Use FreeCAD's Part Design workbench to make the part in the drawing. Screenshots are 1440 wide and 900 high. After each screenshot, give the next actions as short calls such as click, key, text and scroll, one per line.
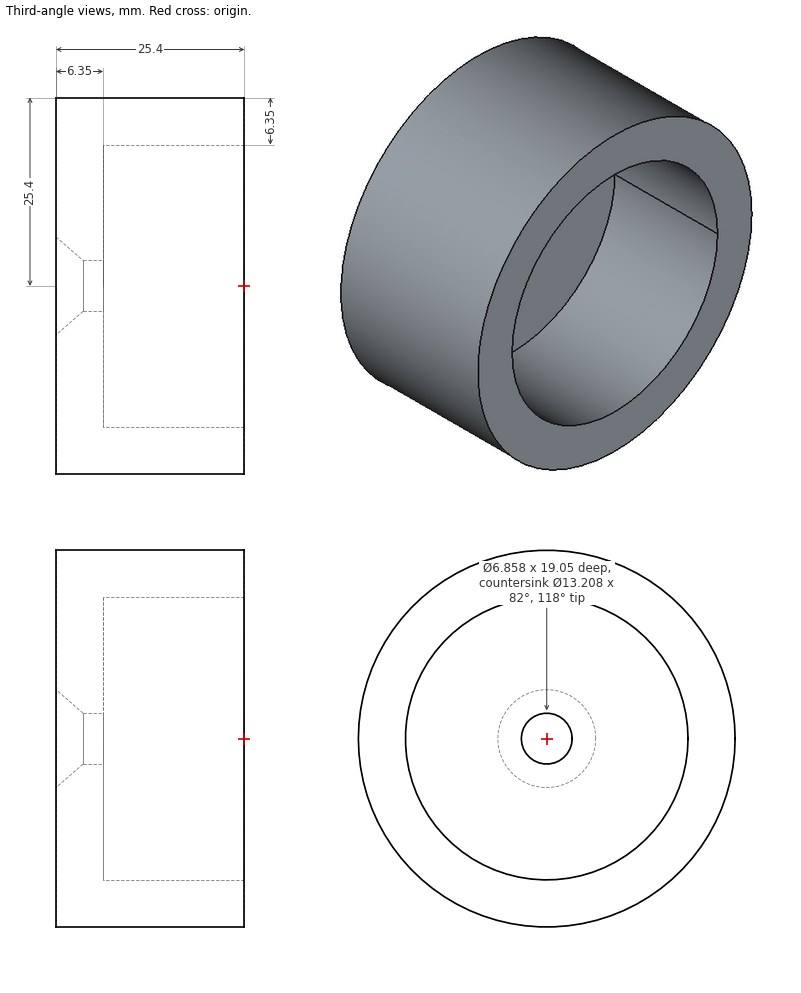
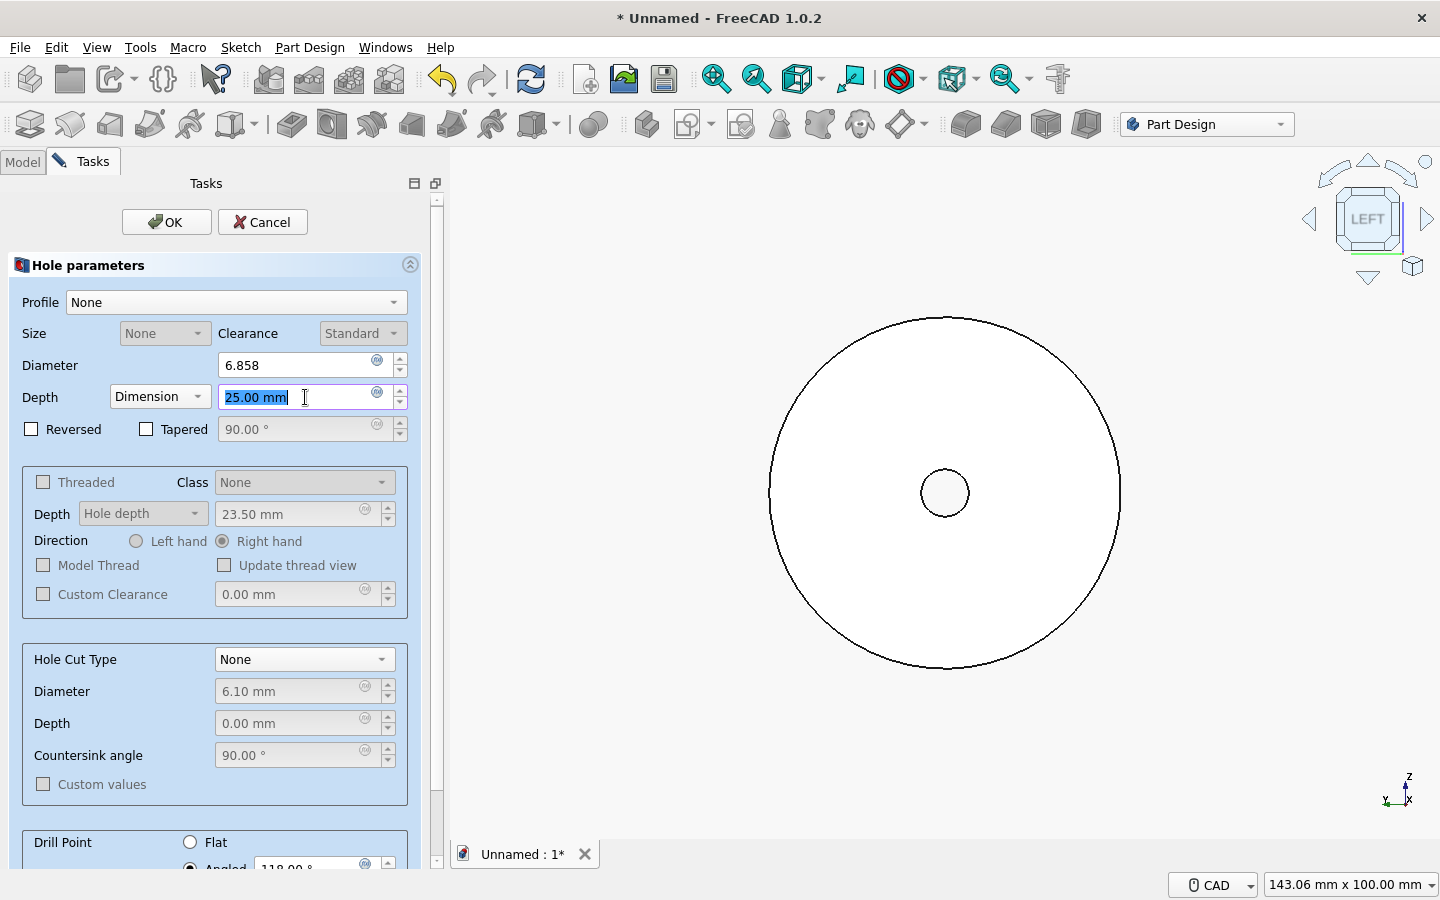
text(19.05)
key(Tab)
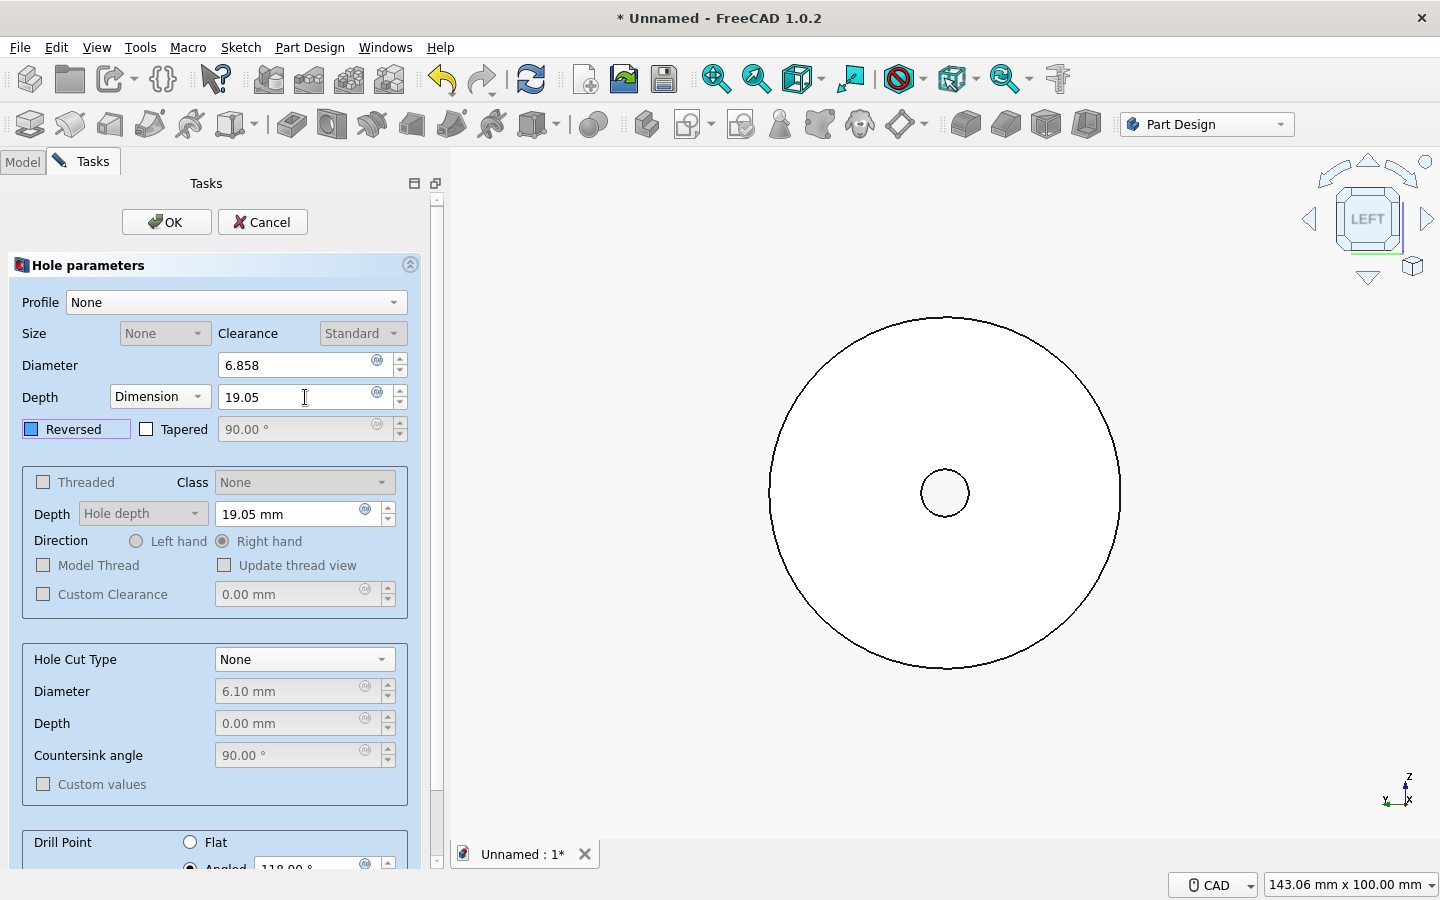
click(306, 660)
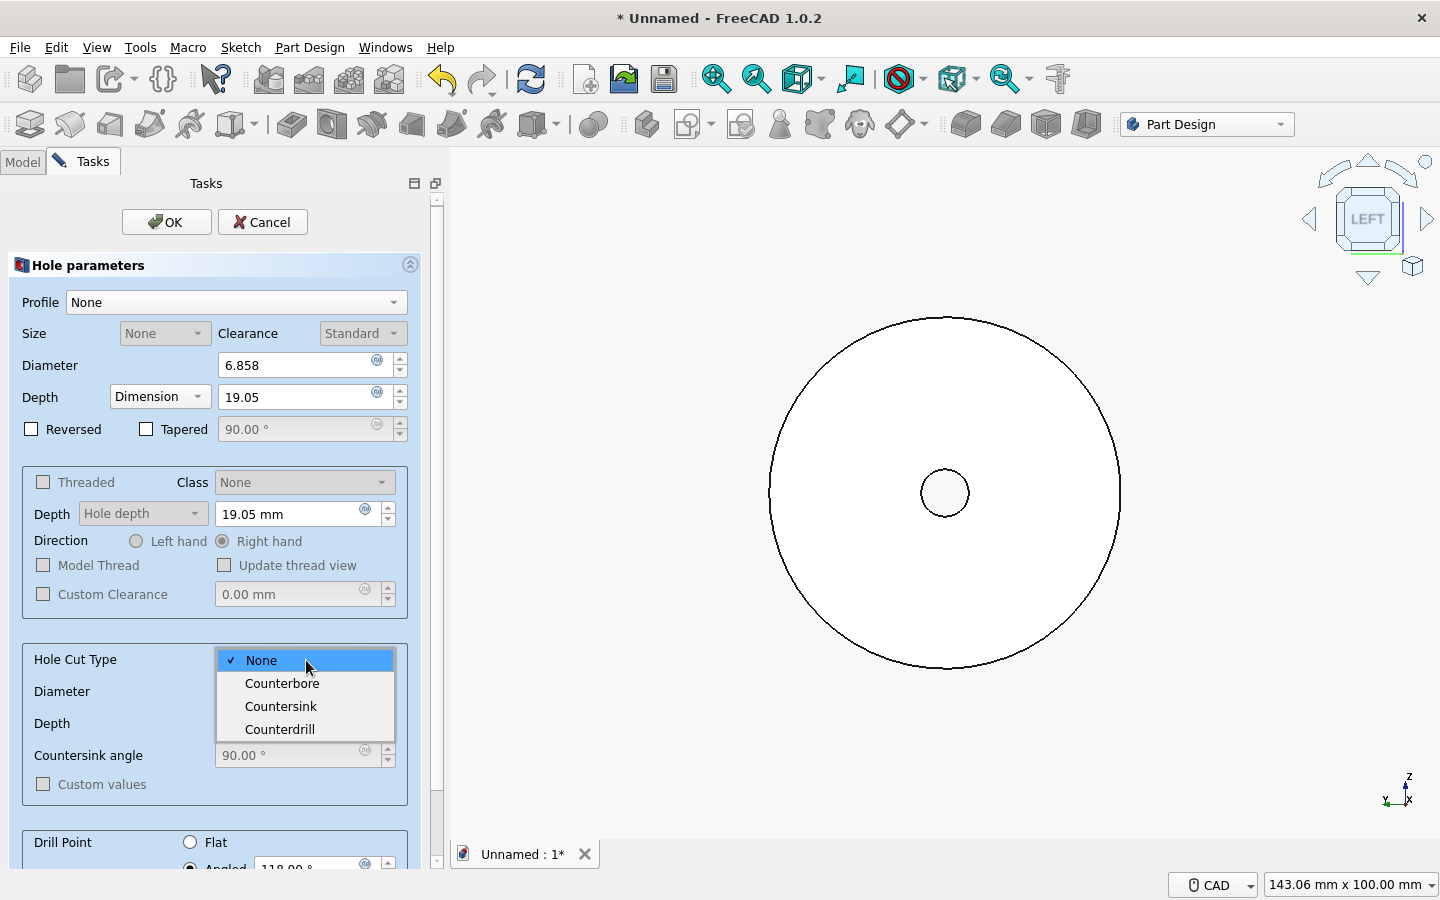
click(304, 706)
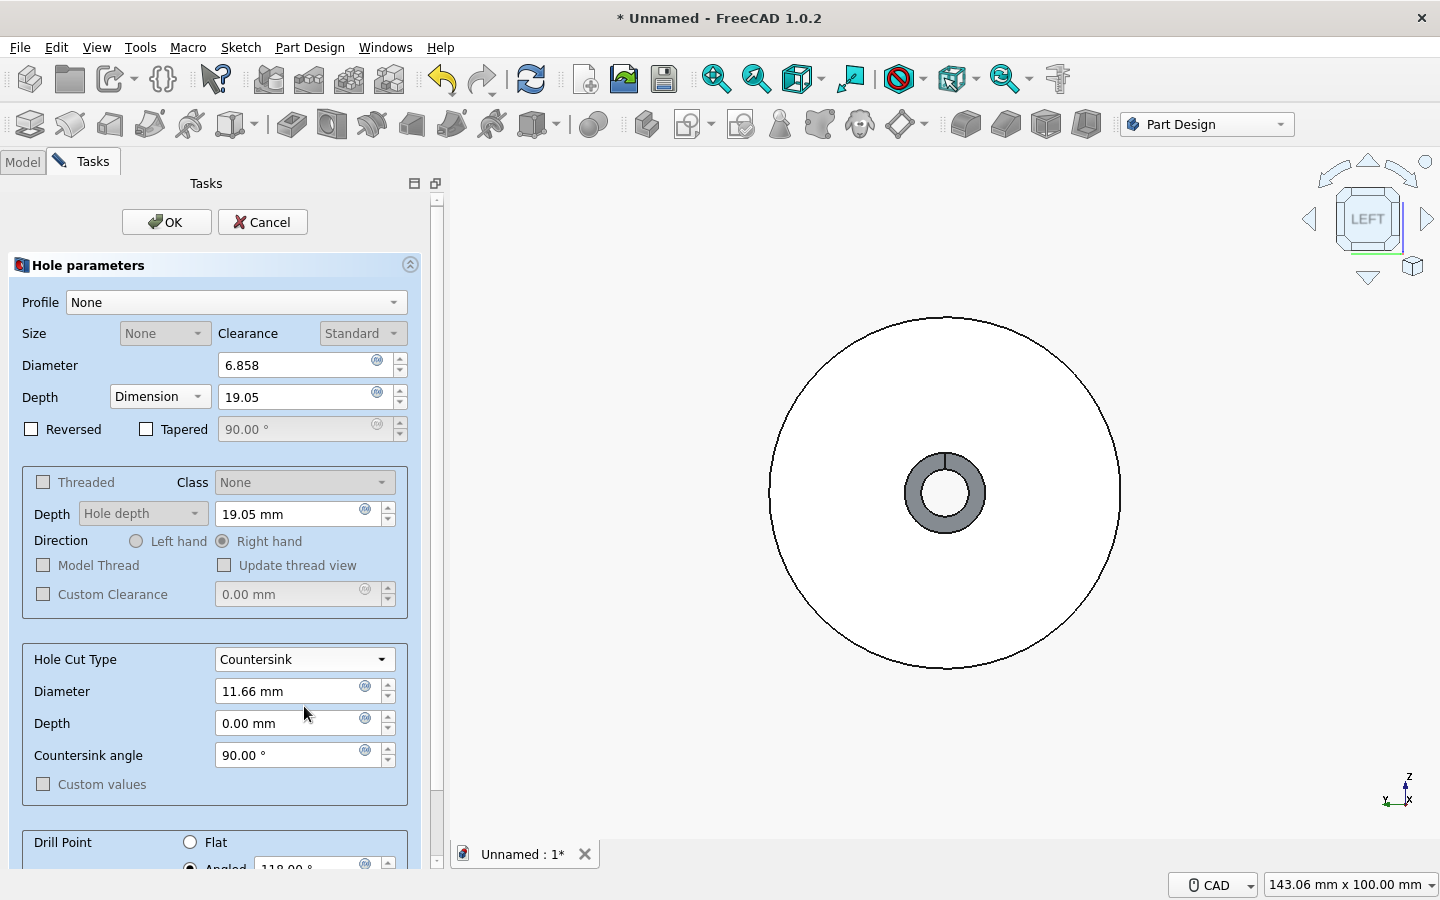
triple_click(298, 755)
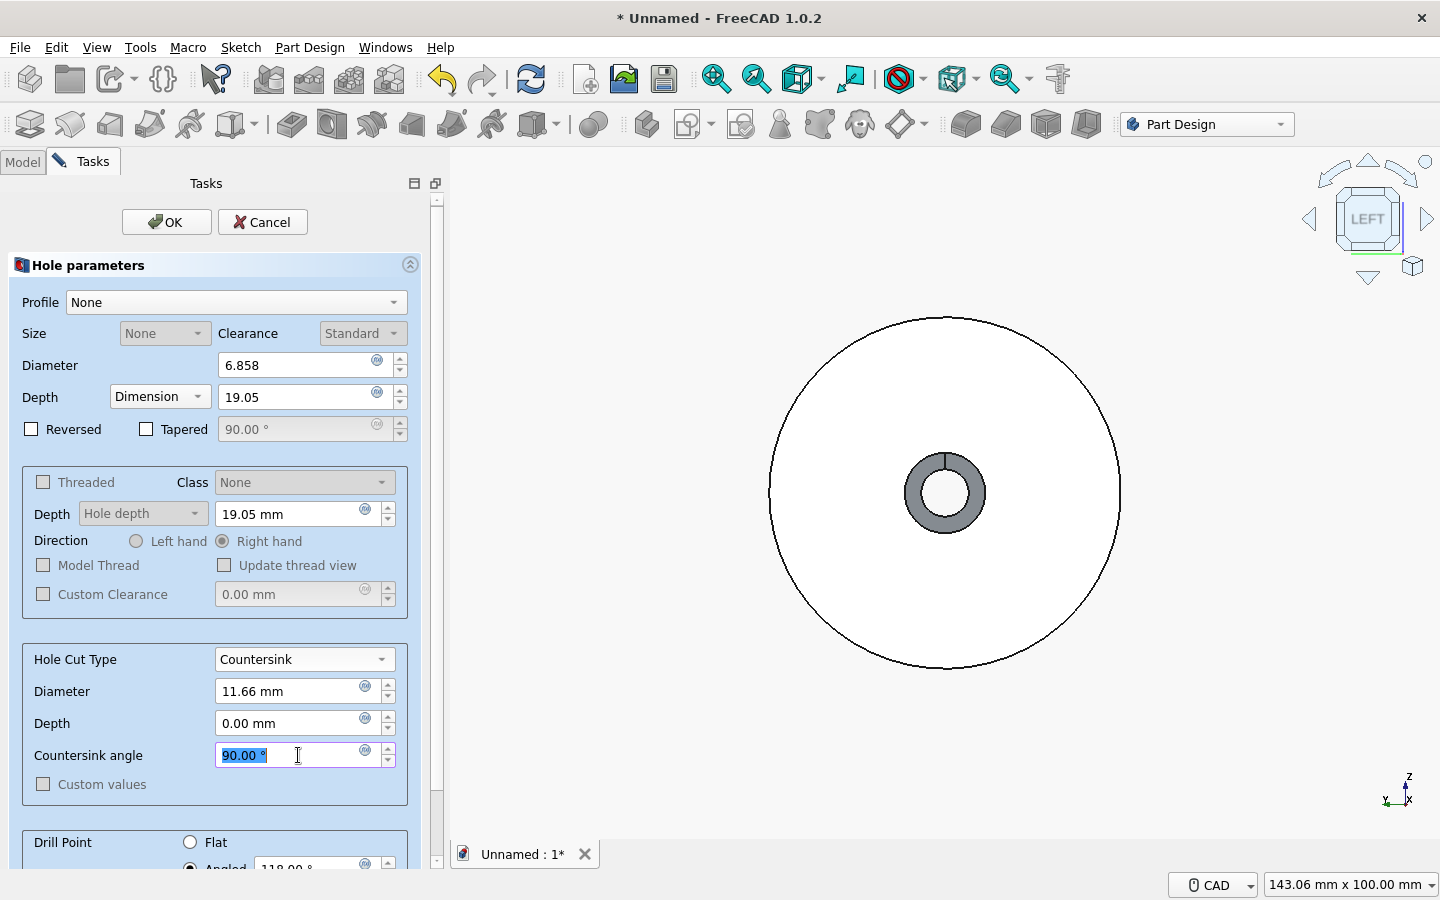
text(82)
key(Tab)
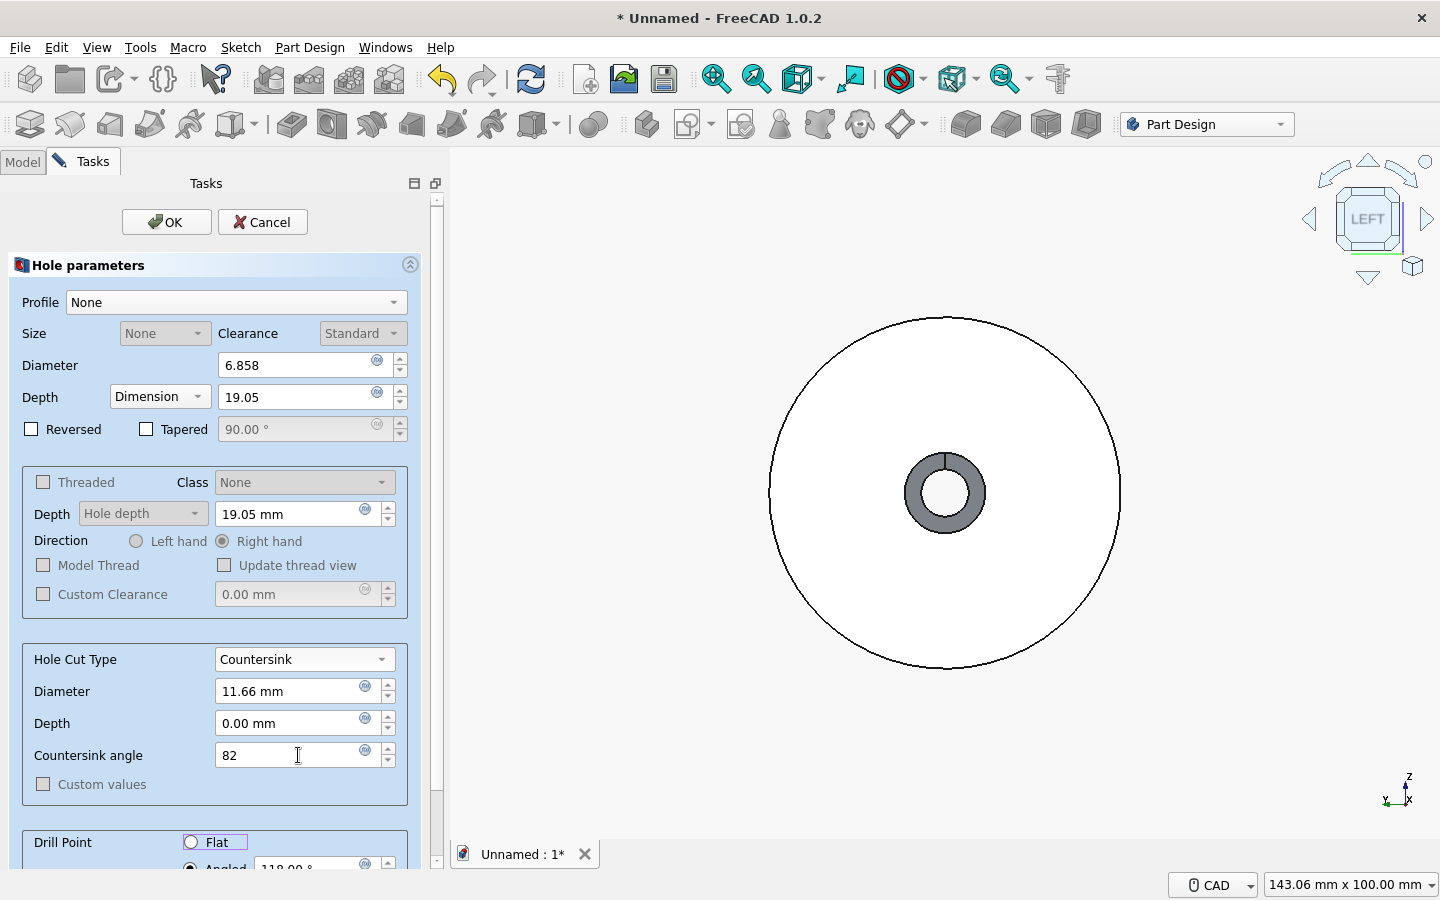
triple_click(298, 691)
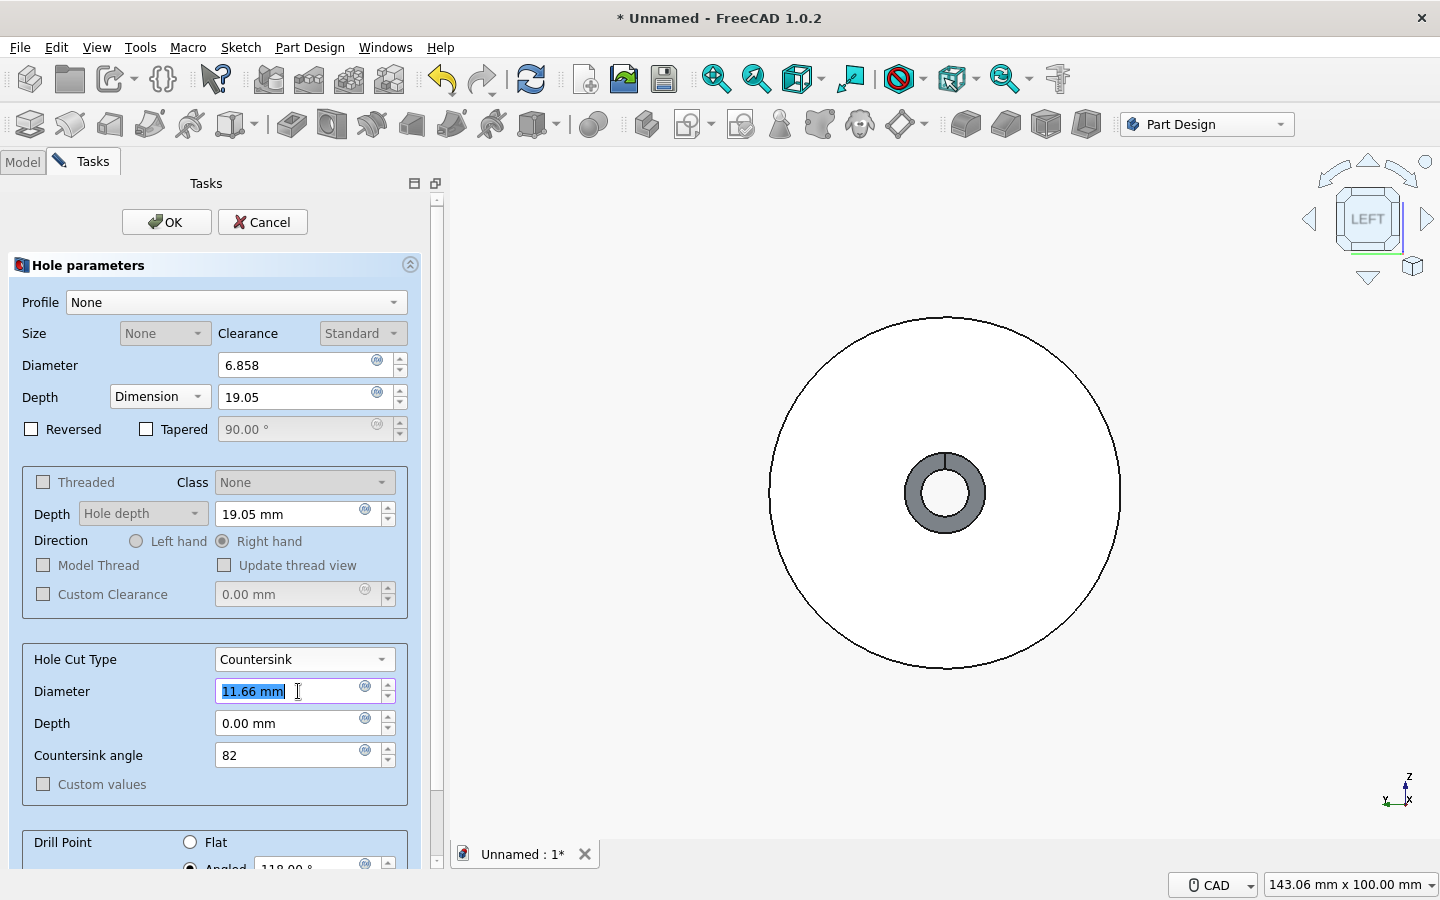
text(13.208)
key(Tab)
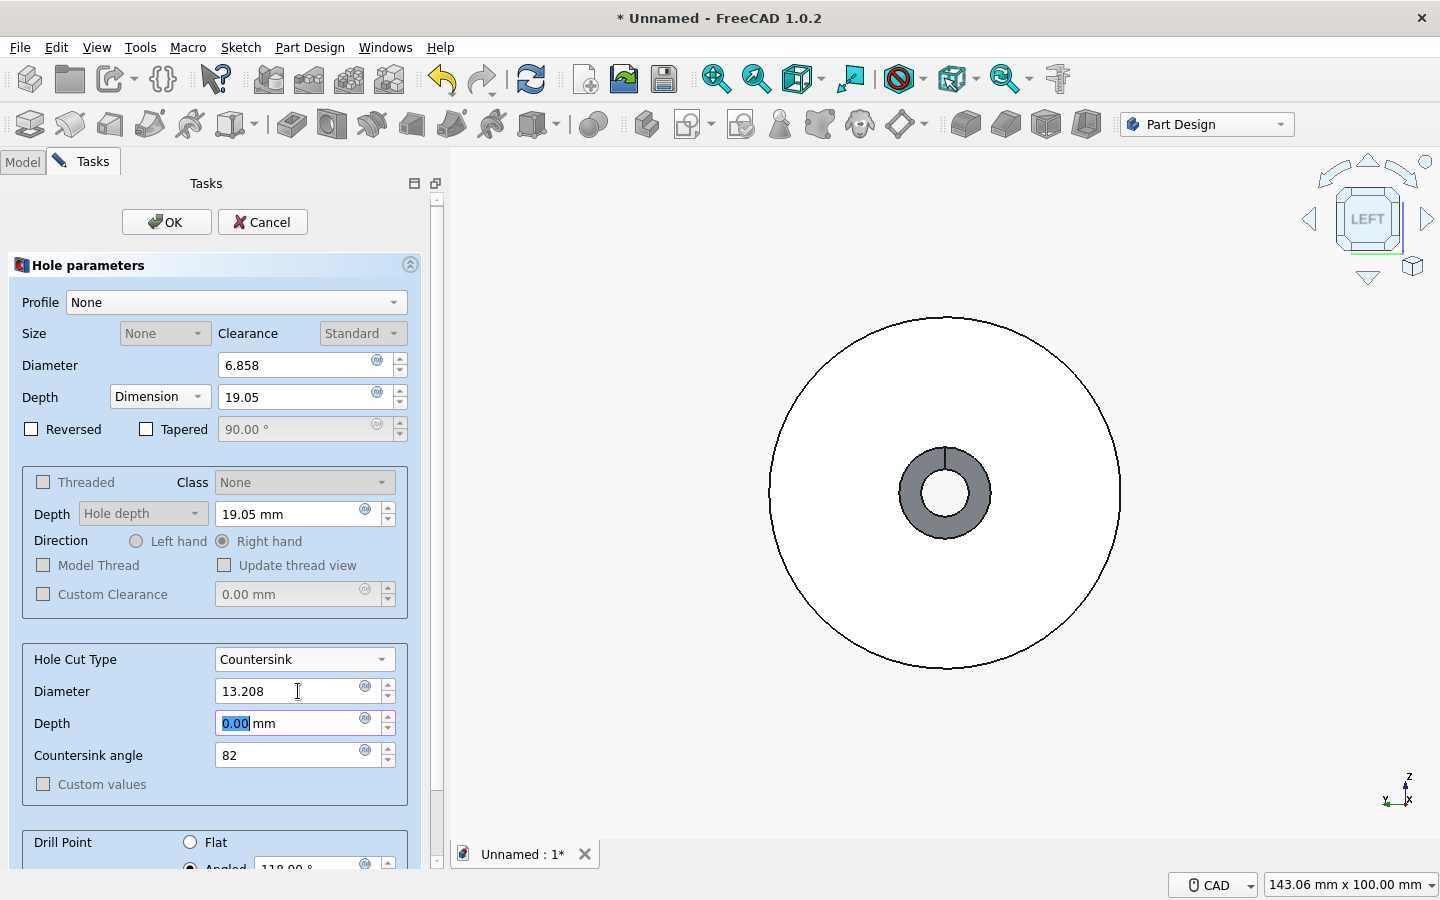
click(167, 222)